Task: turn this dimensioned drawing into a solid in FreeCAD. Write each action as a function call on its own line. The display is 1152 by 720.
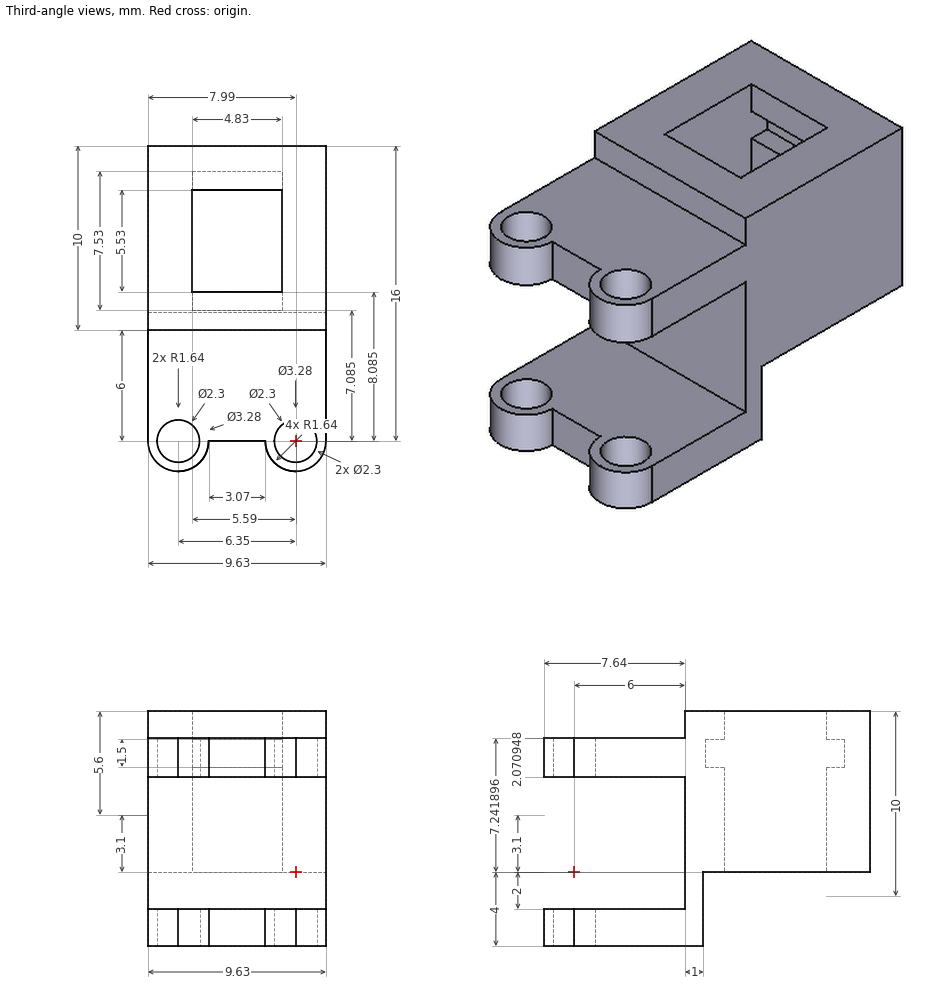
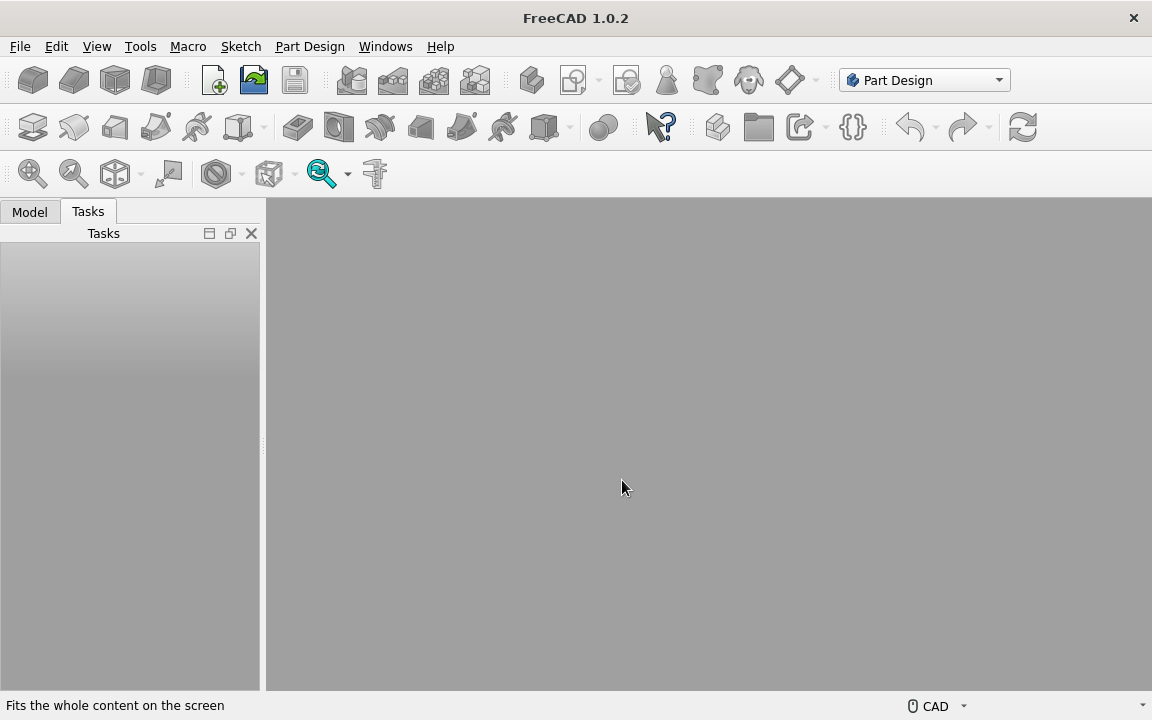
click(213, 80)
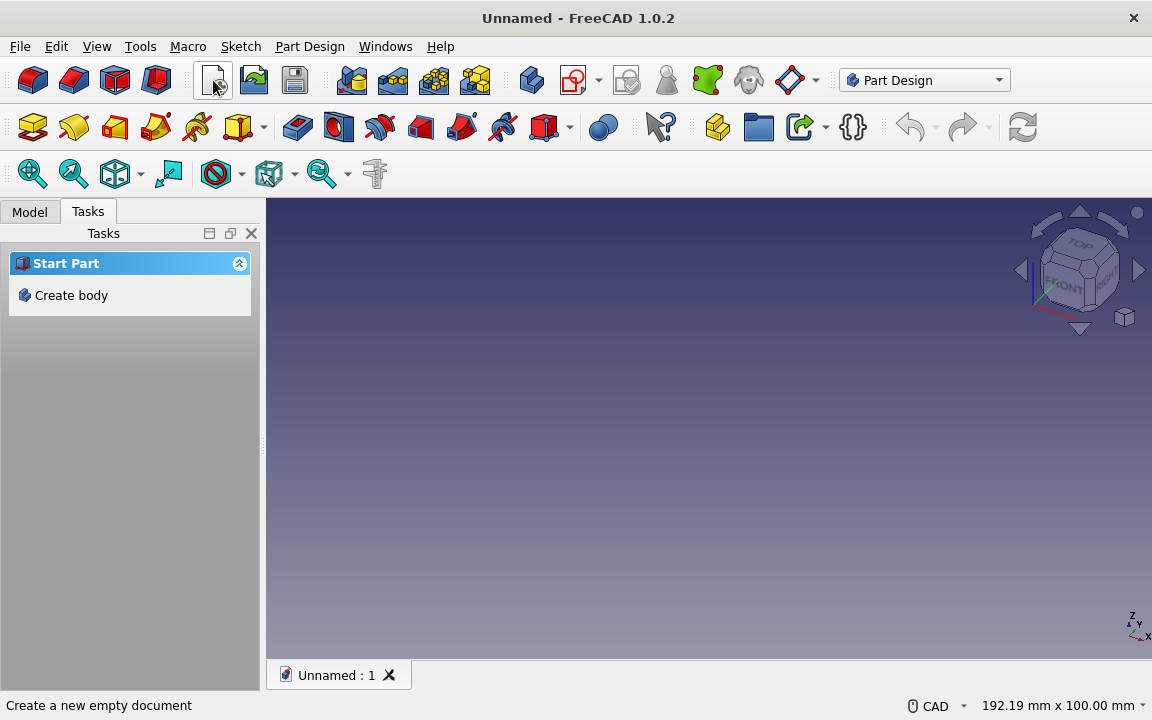
click(572, 80)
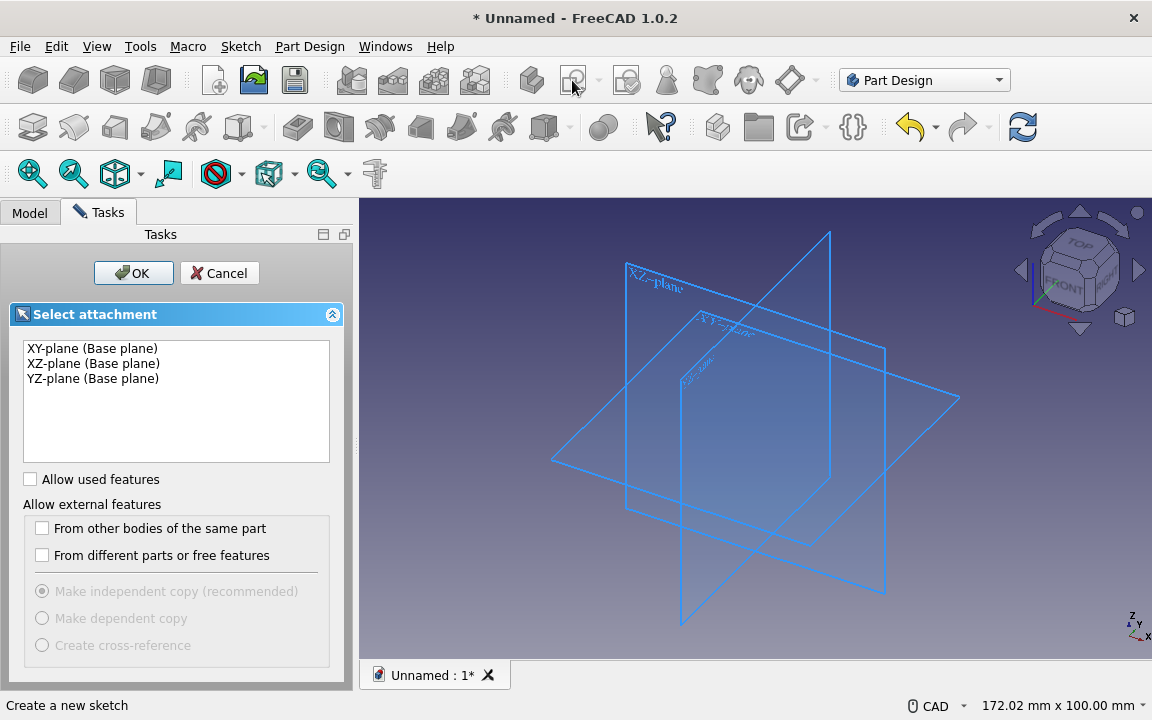
click(84, 348)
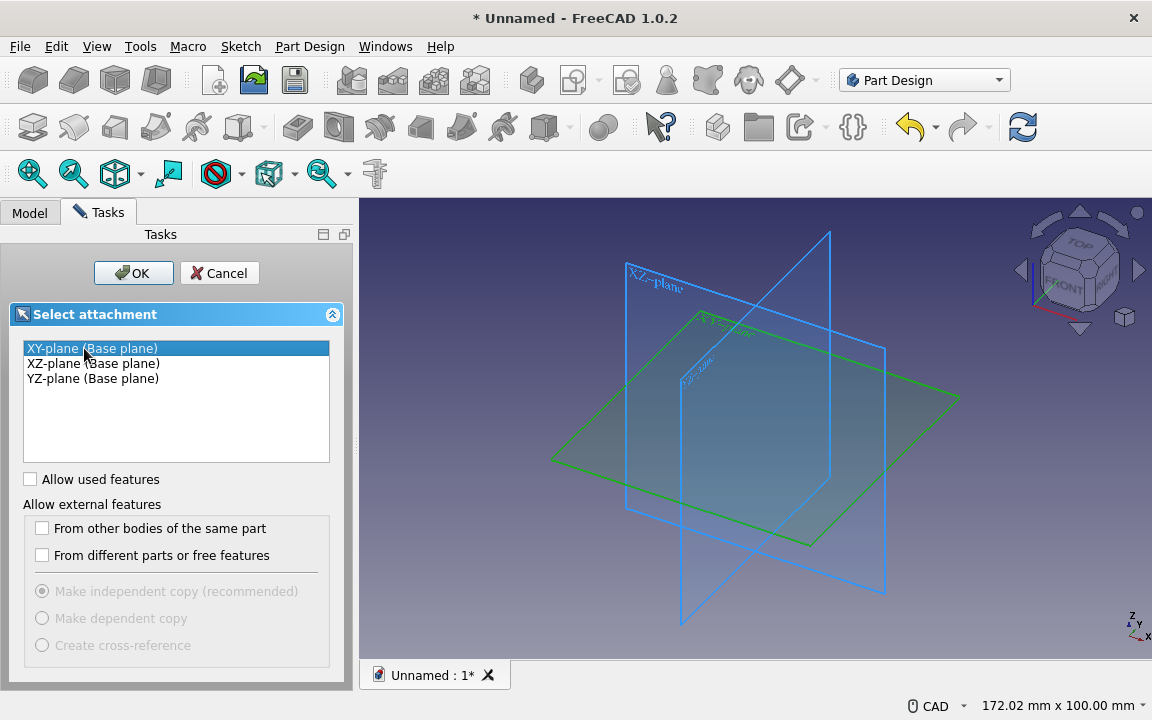
click(134, 273)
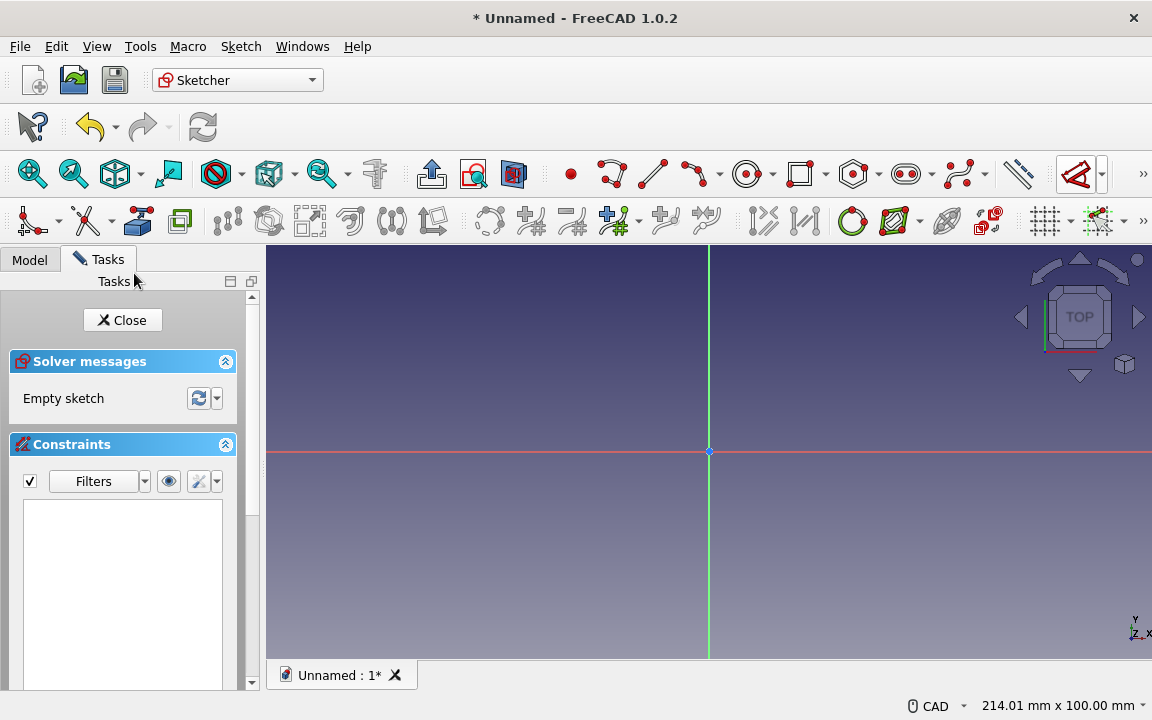
scroll(713, 452, up, 15)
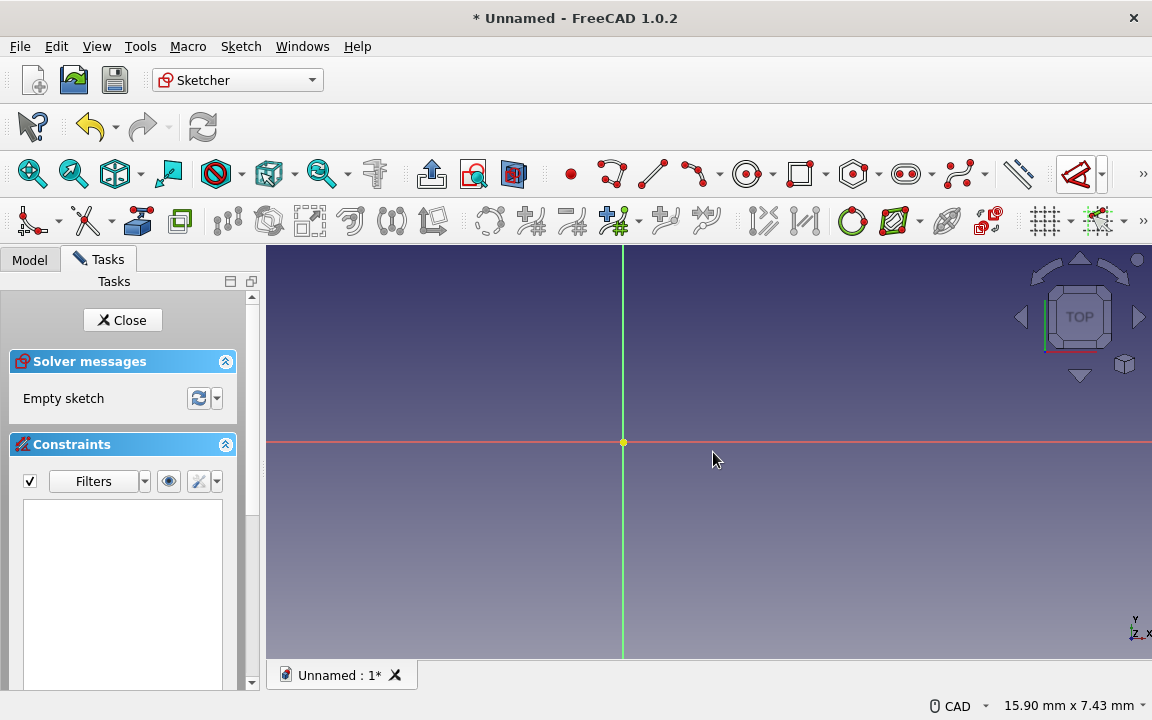
click(746, 174)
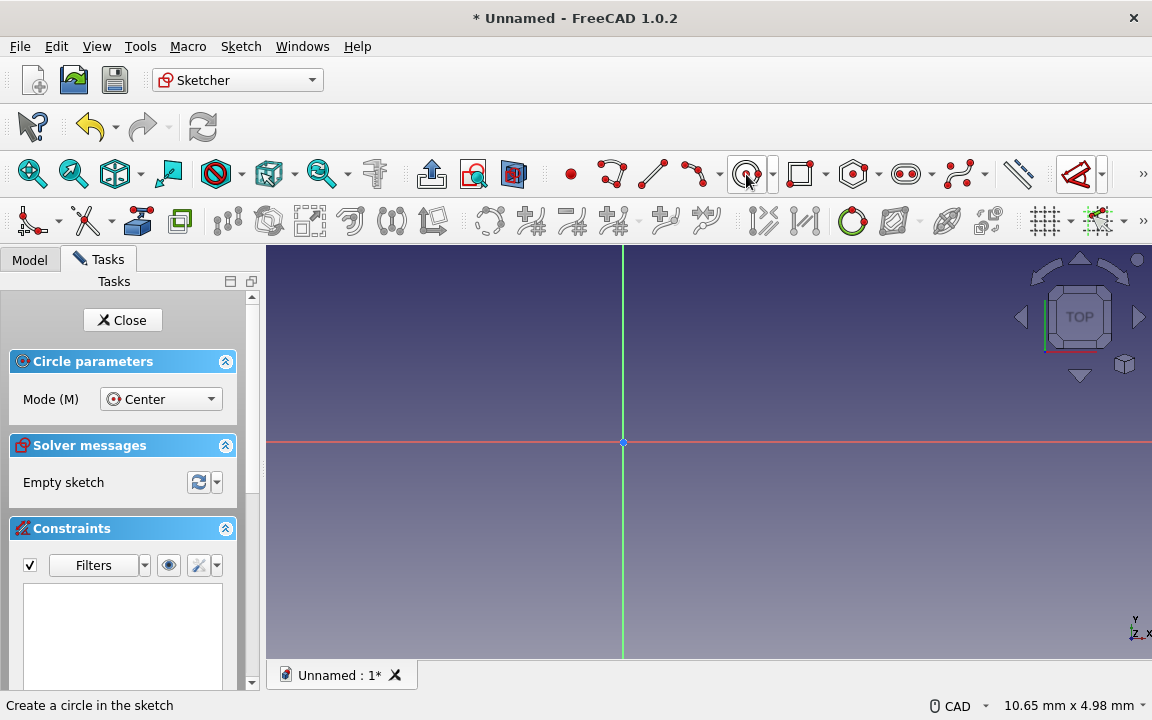
click(623, 442)
click(719, 346)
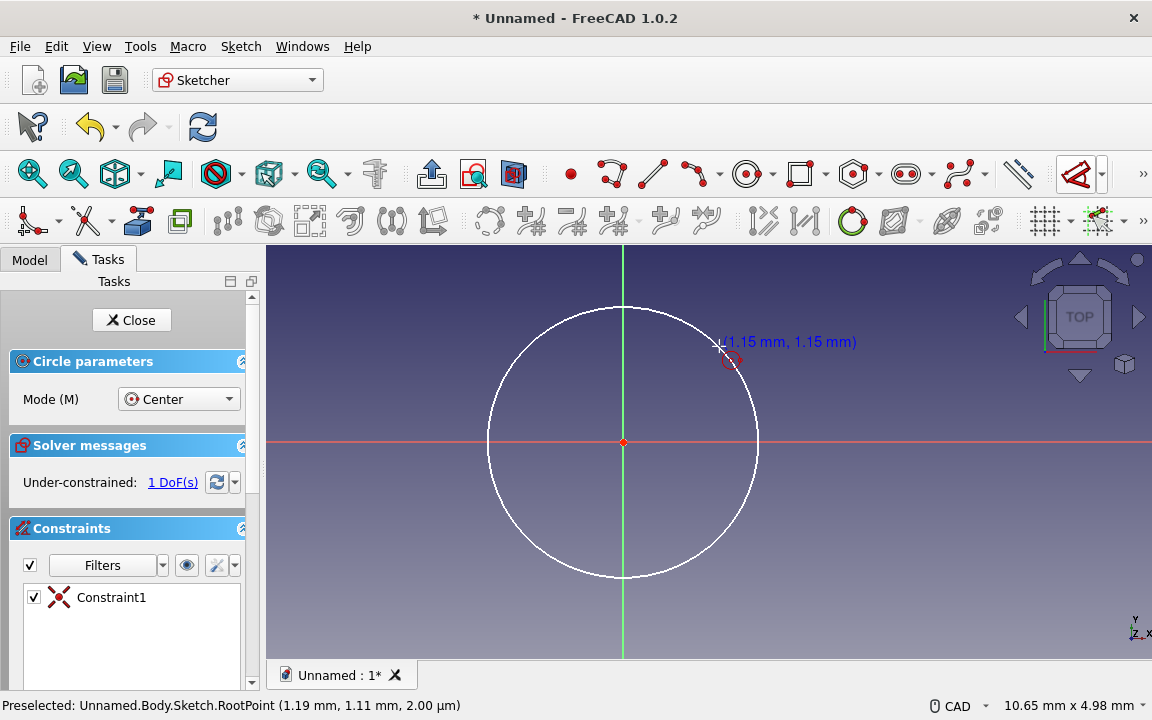
click(623, 442)
click(691, 375)
key(Escape)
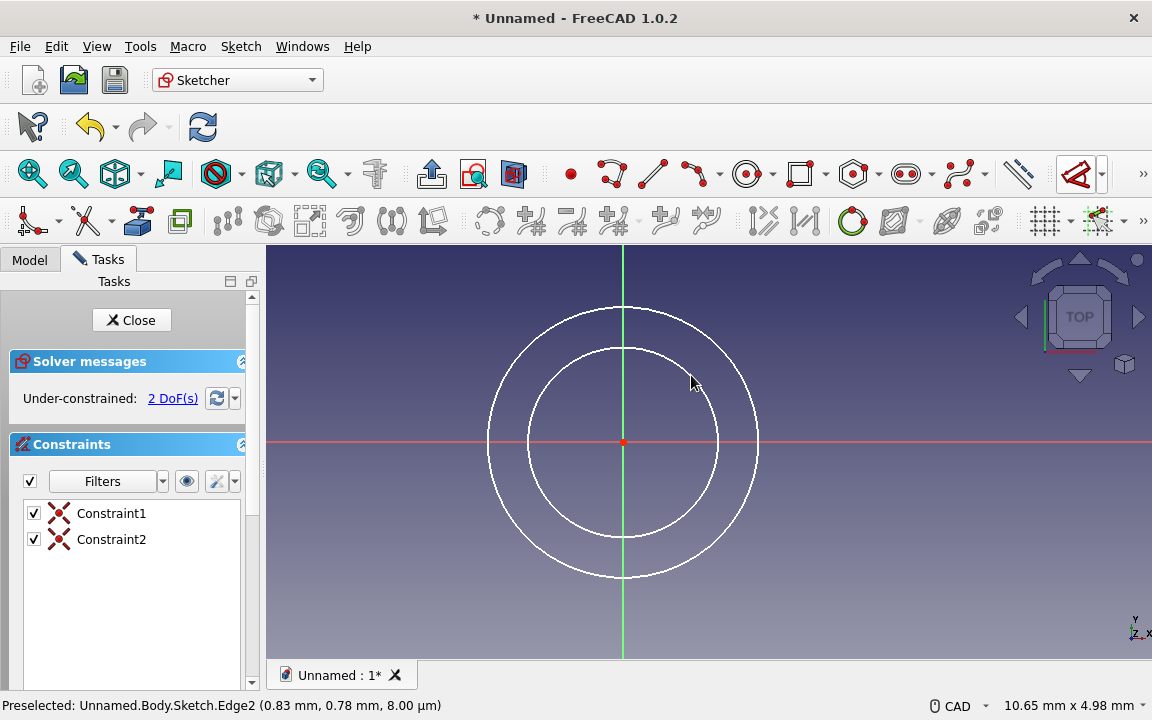
key(d)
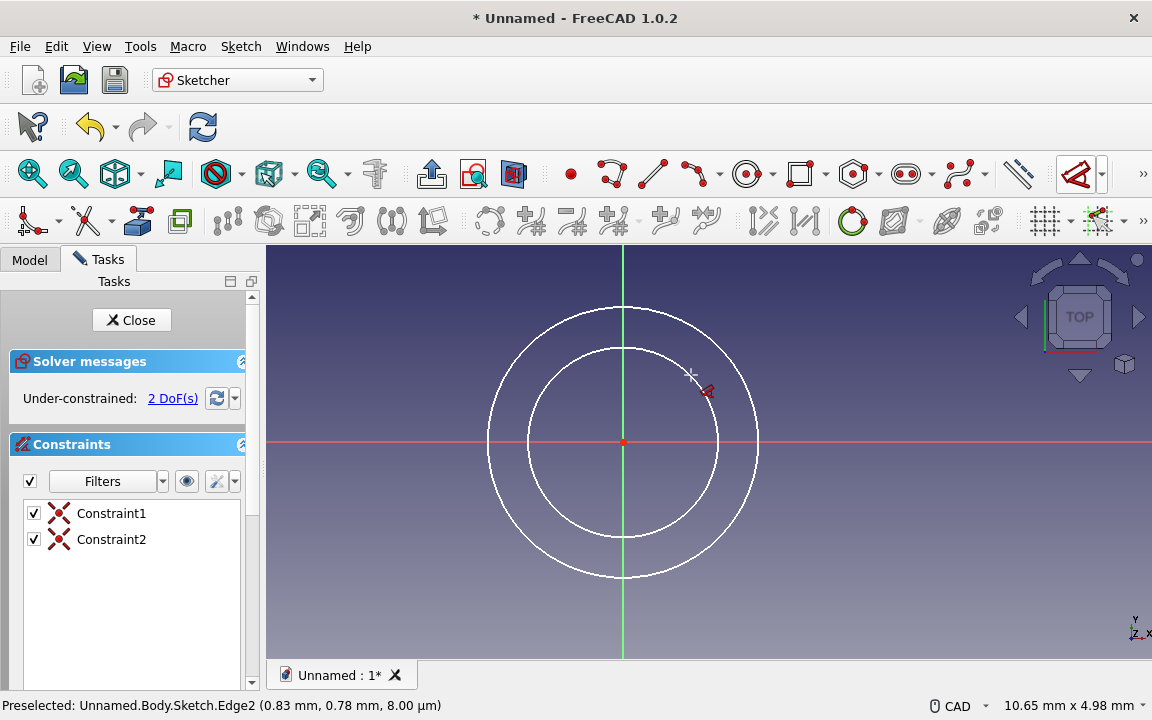
click(718, 346)
click(740, 323)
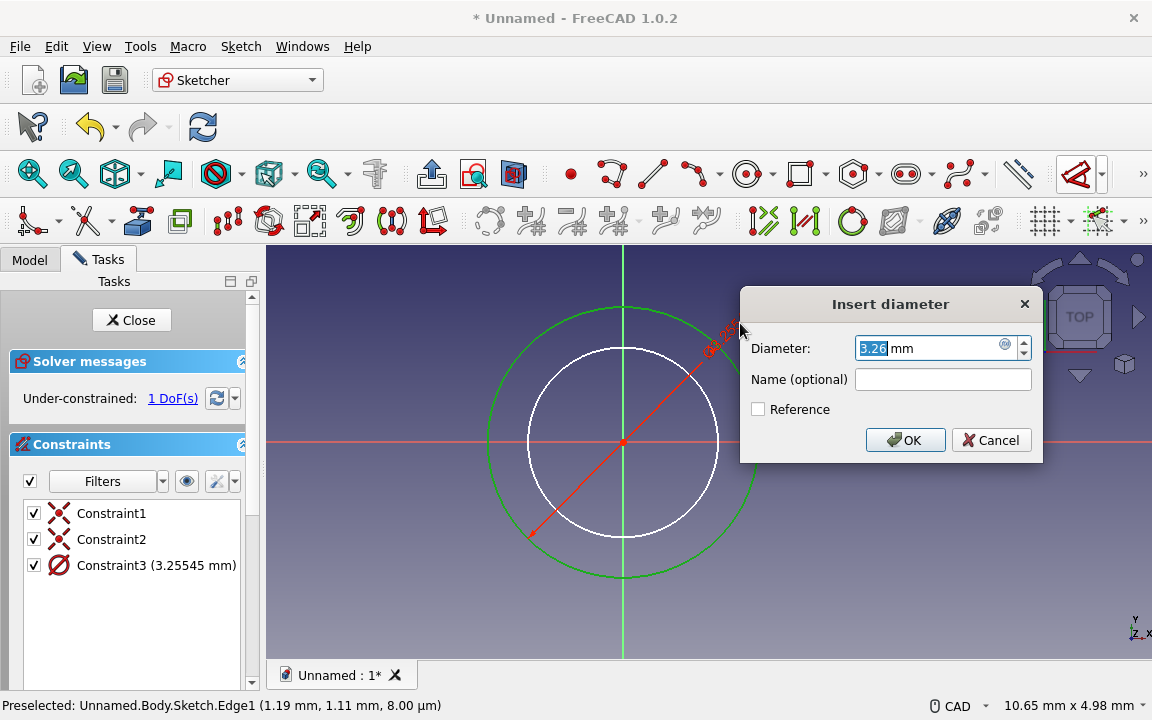
text(3.28)
key(Return)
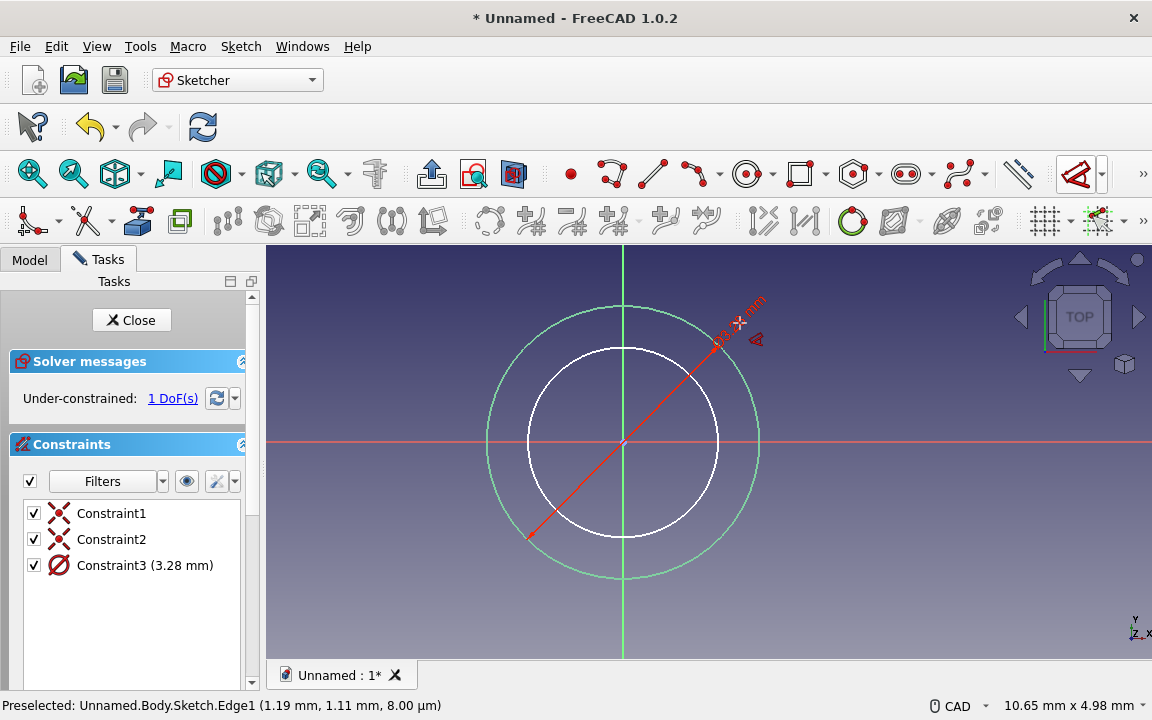
click(690, 375)
click(767, 400)